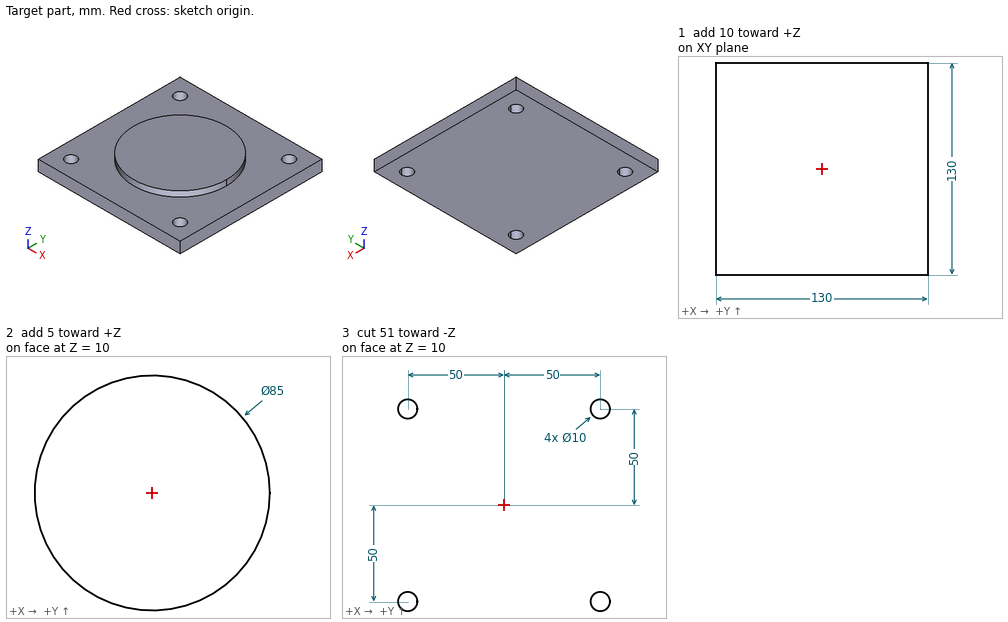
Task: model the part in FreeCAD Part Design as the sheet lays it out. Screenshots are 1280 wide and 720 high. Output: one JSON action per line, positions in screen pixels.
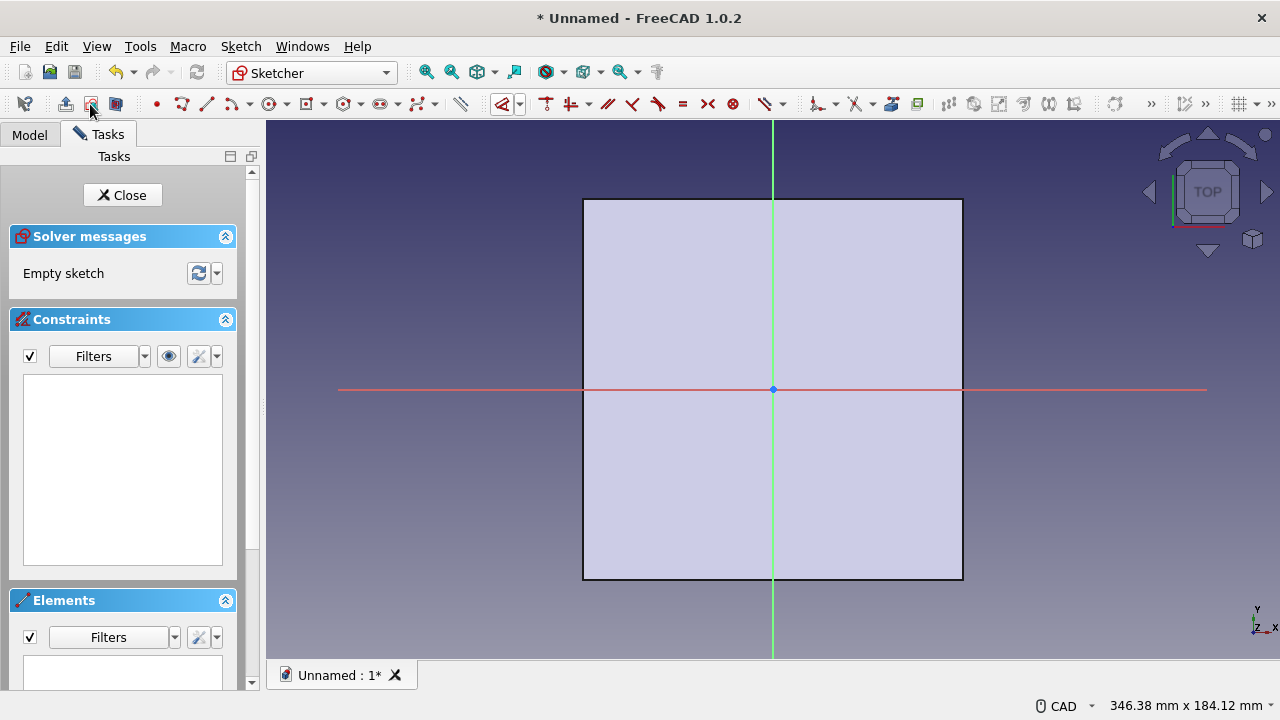
{"action": "scroll", "coordinate": [912, 390], "scroll_direction": "up", "scroll_amount": 2}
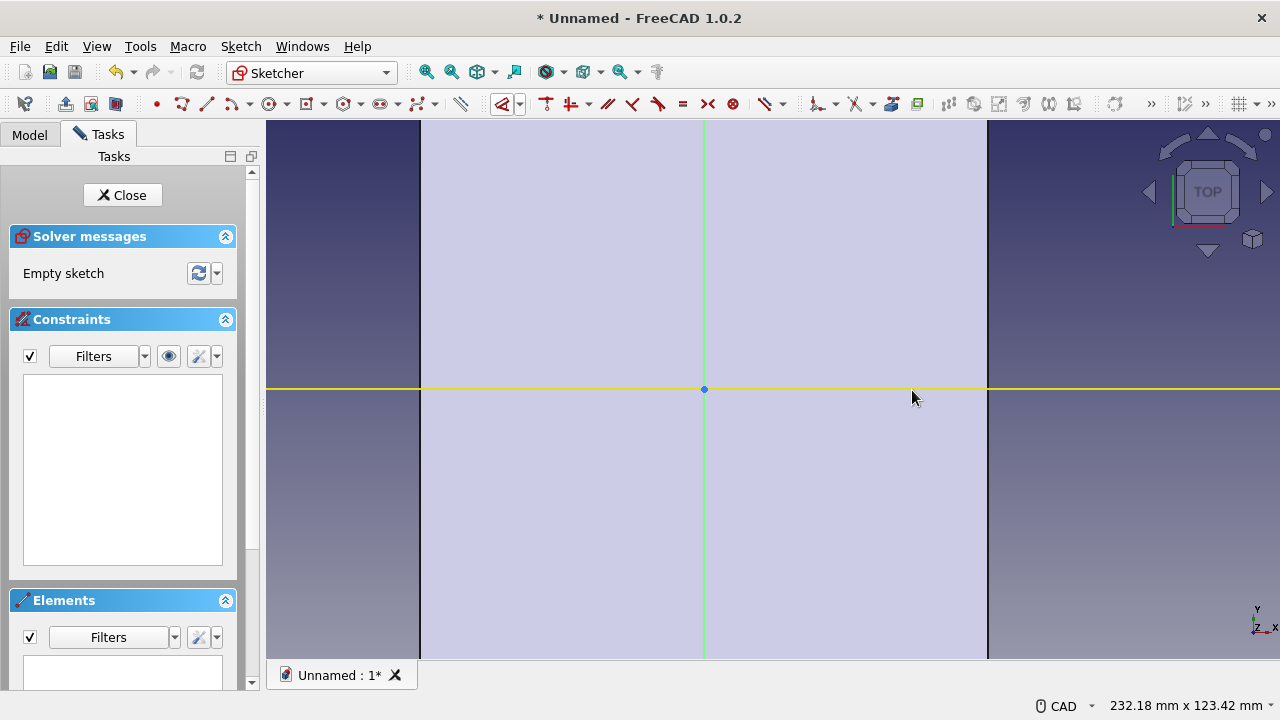
{"action": "left_click", "coordinate": [268, 104]}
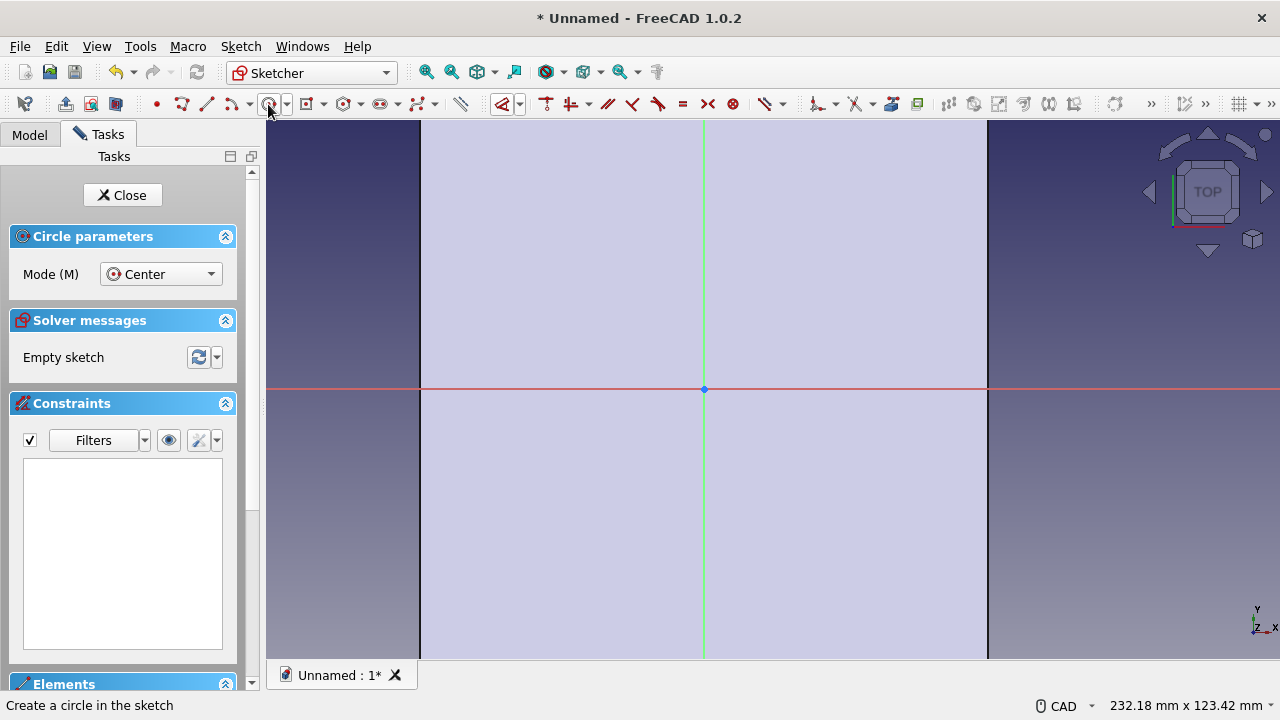
{"action": "left_click", "coordinate": [704, 389]}
{"action": "left_click", "coordinate": [836, 258]}
{"action": "key", "text": "Escape"}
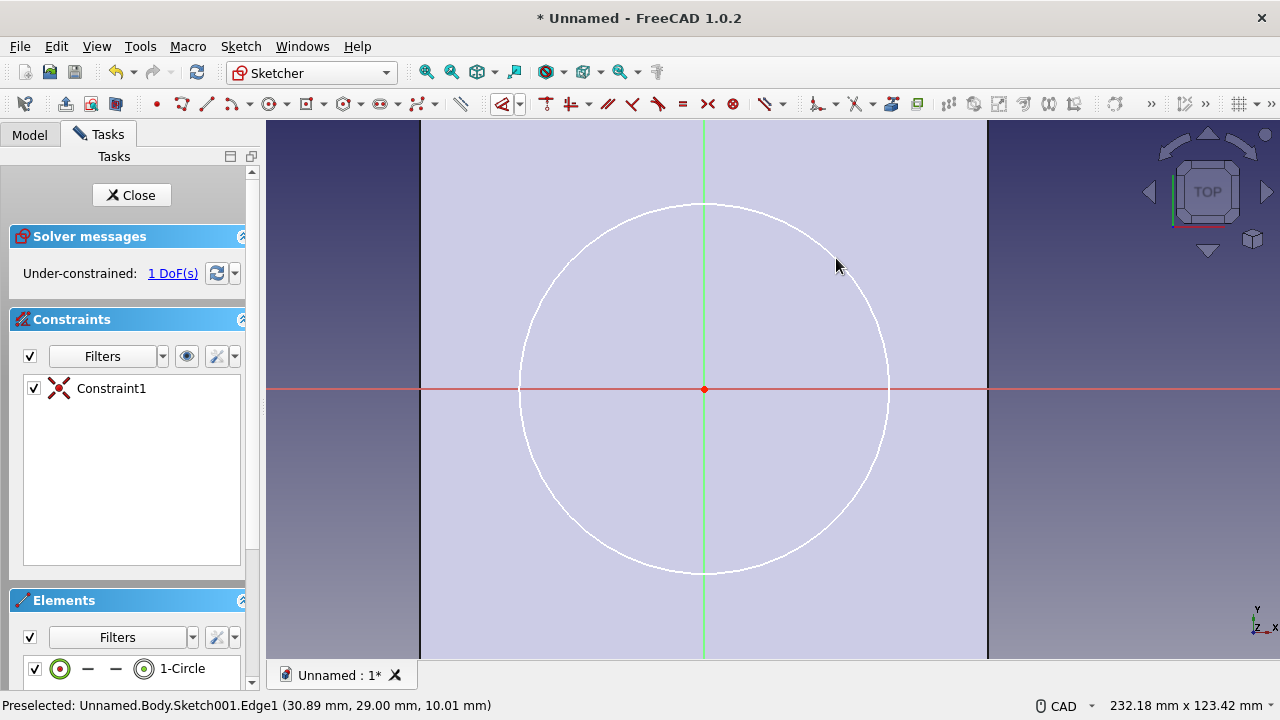
{"action": "left_click", "coordinate": [835, 258]}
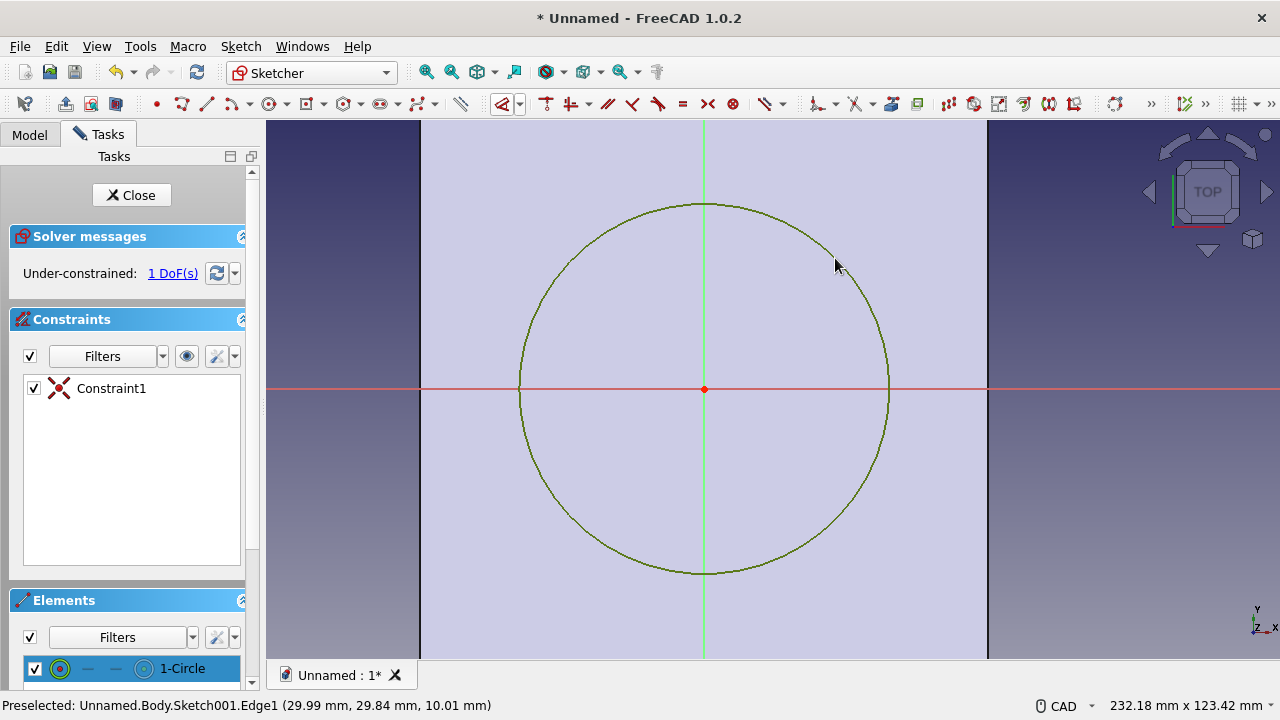
{"action": "left_click", "coordinate": [520, 104]}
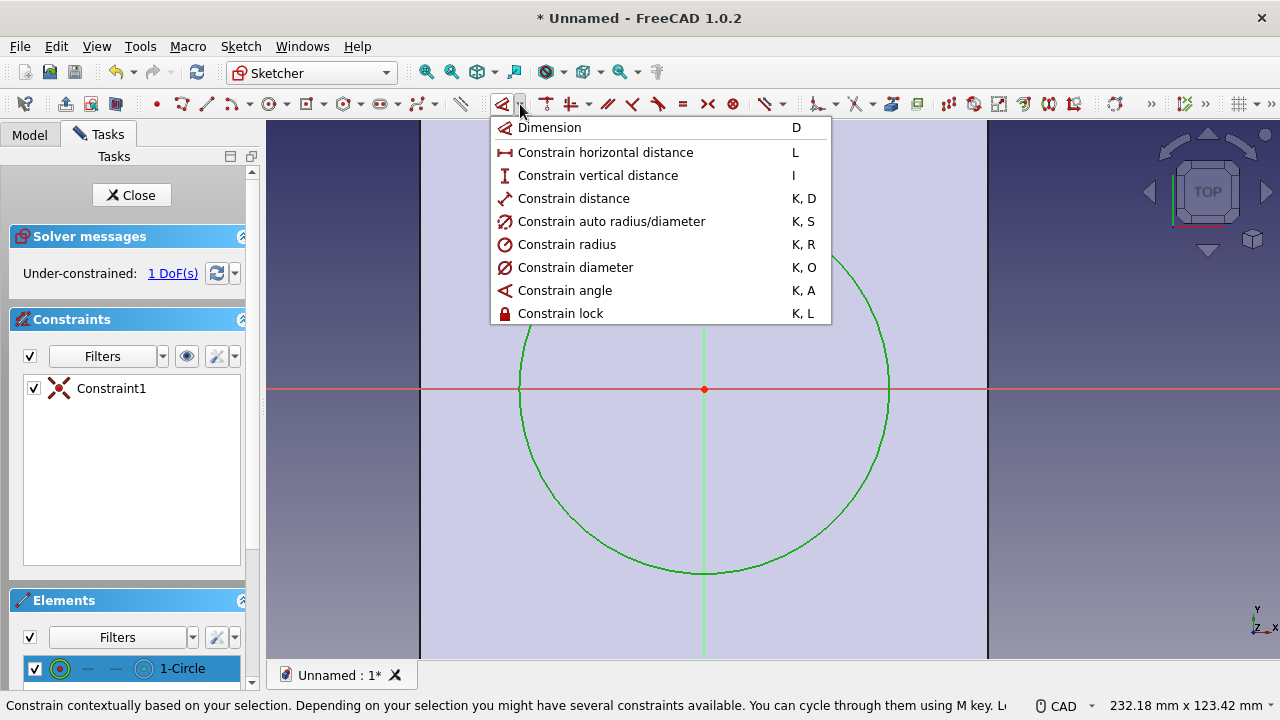
{"action": "left_click", "coordinate": [661, 268]}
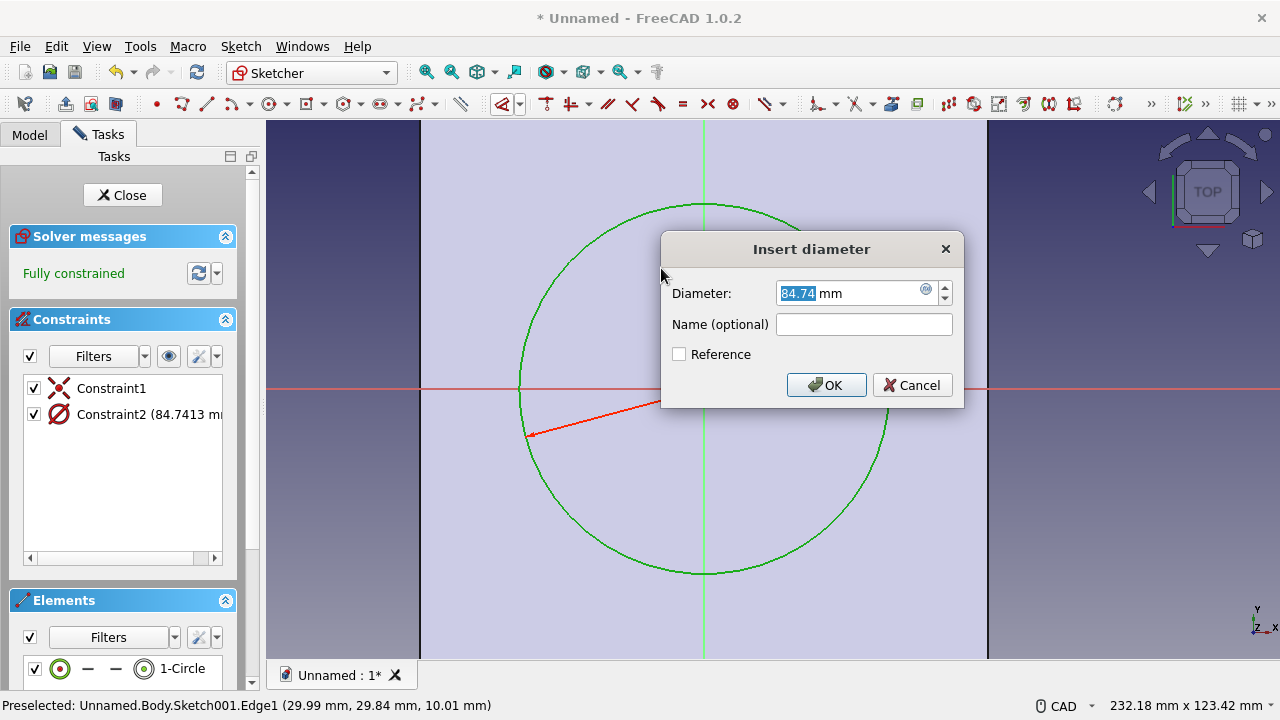
{"action": "type", "text": "85"}
{"action": "key", "text": "Return"}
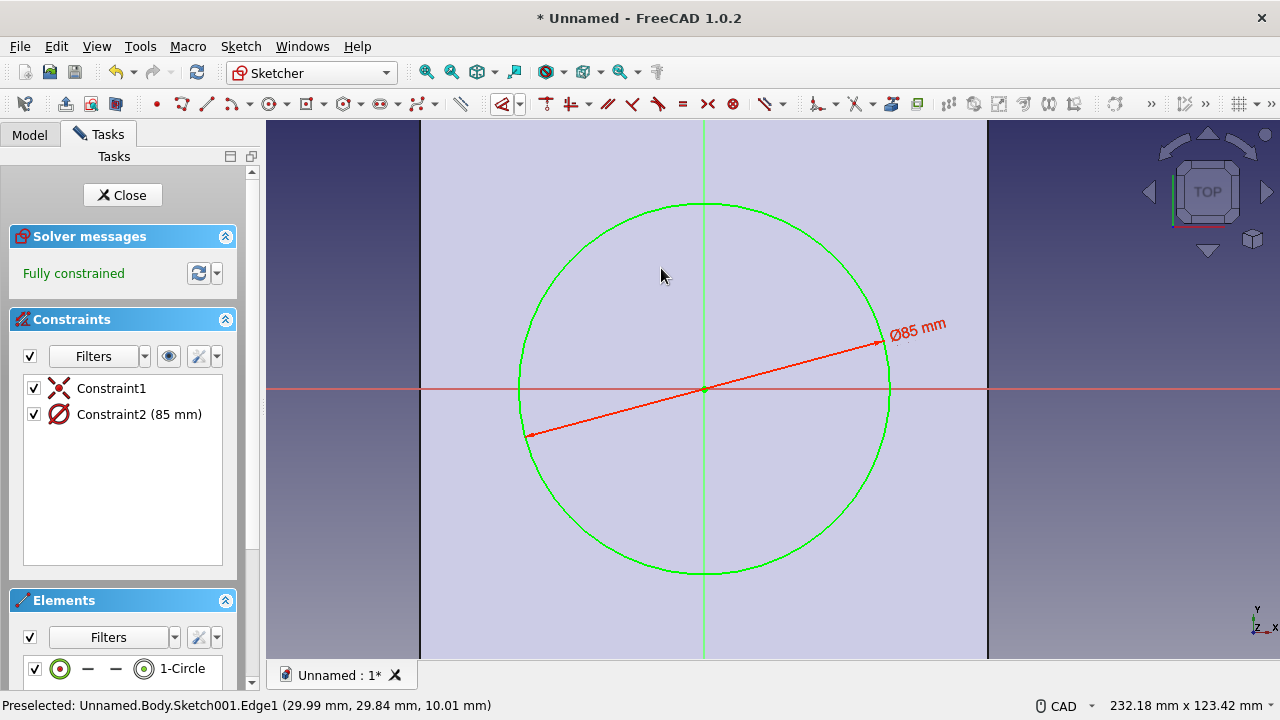
{"action": "left_click", "coordinate": [123, 195]}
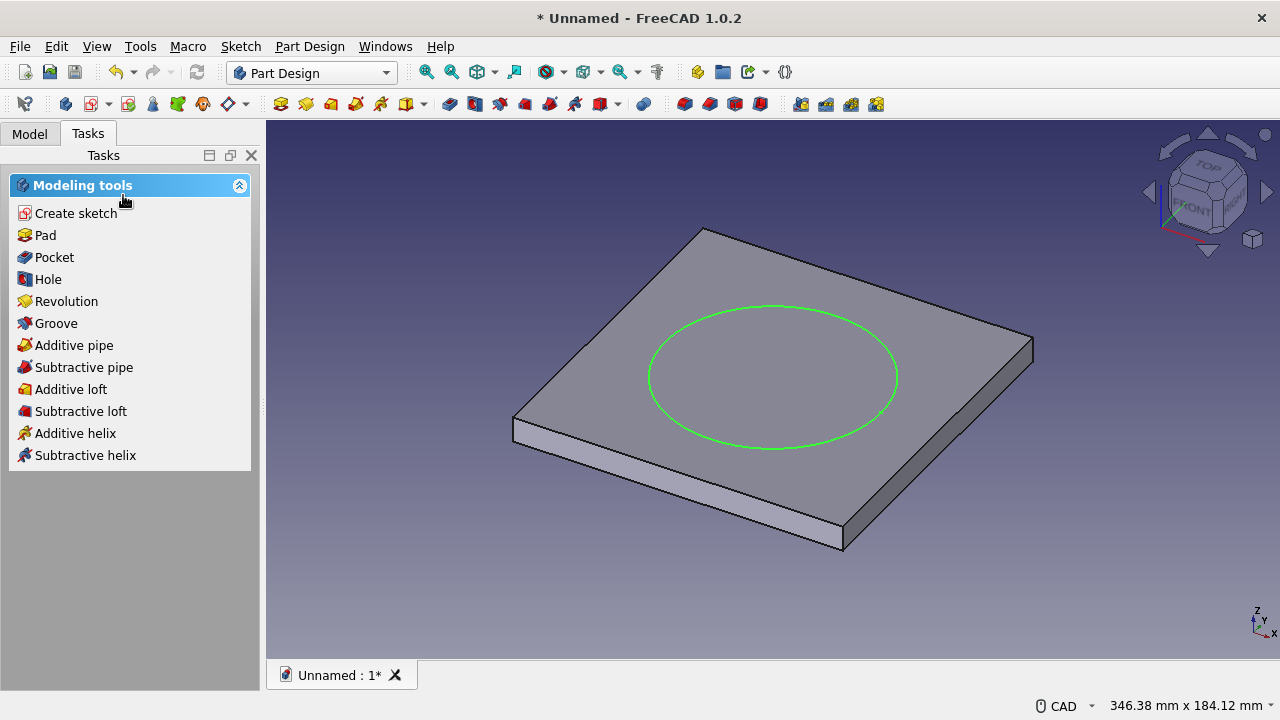
{"action": "left_click", "coordinate": [281, 104]}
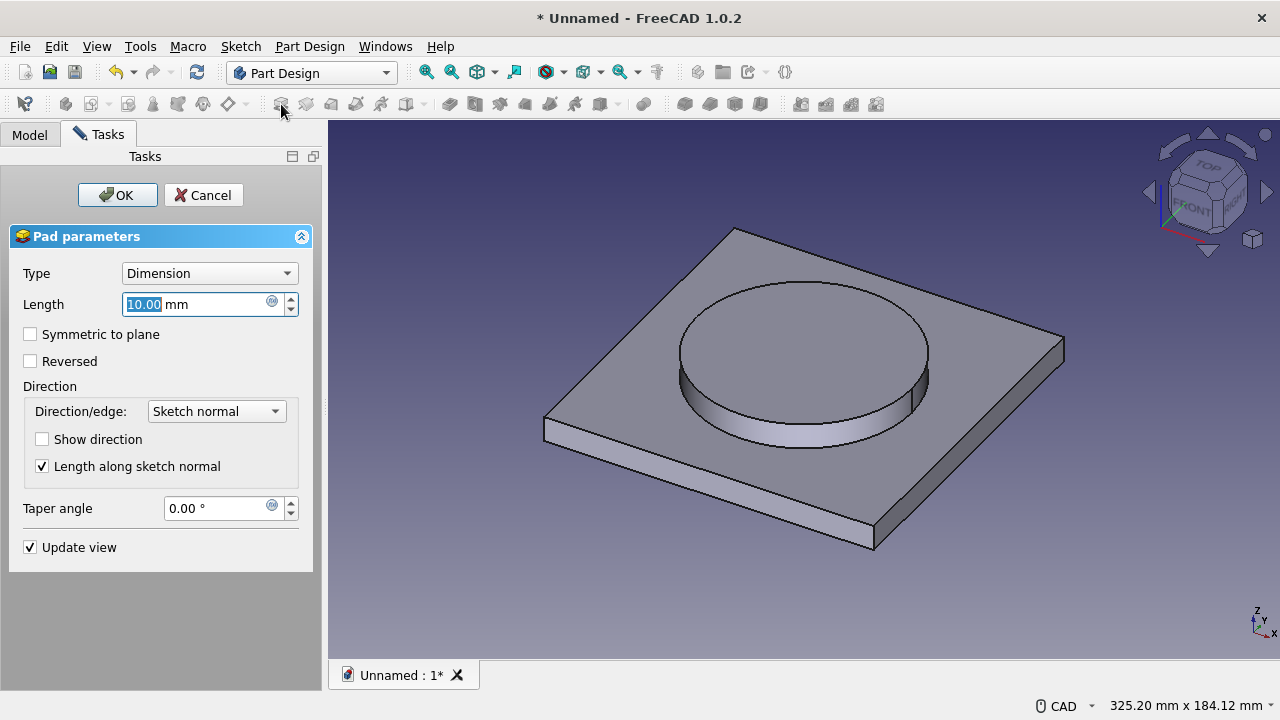
{"action": "type", "text": "5"}
{"action": "key", "text": "Tab"}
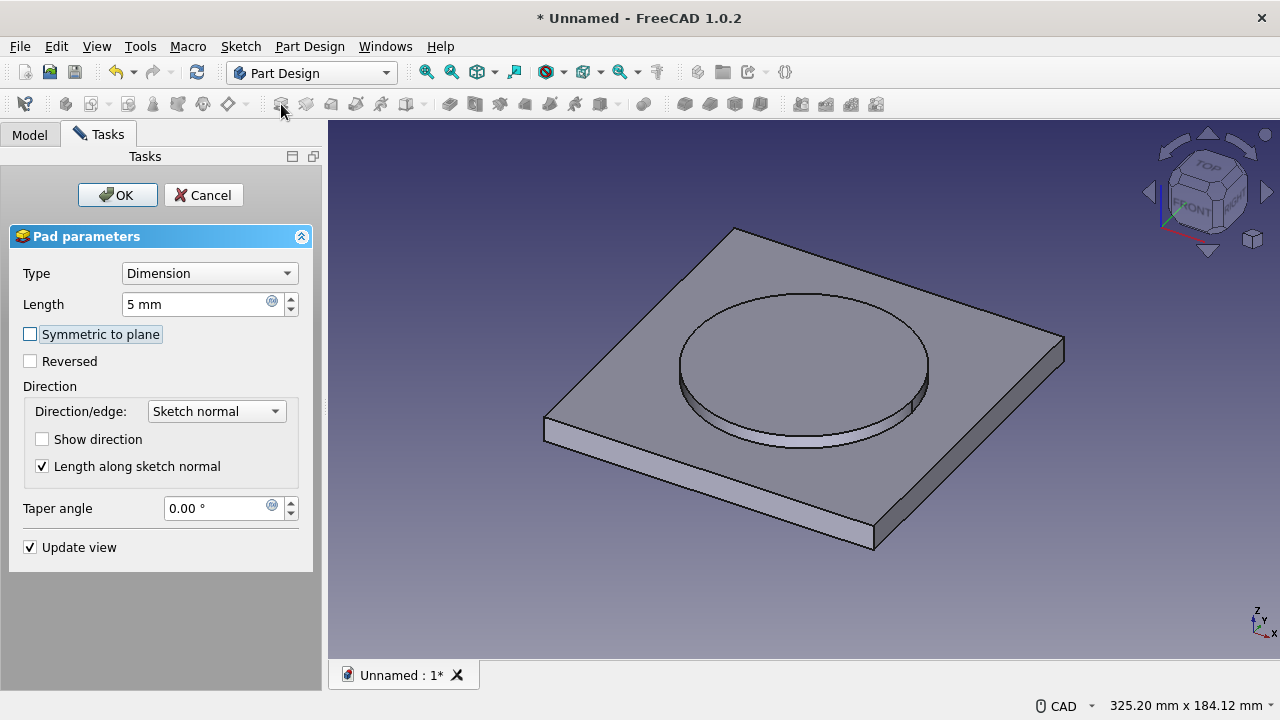
{"action": "left_click", "coordinate": [118, 195]}